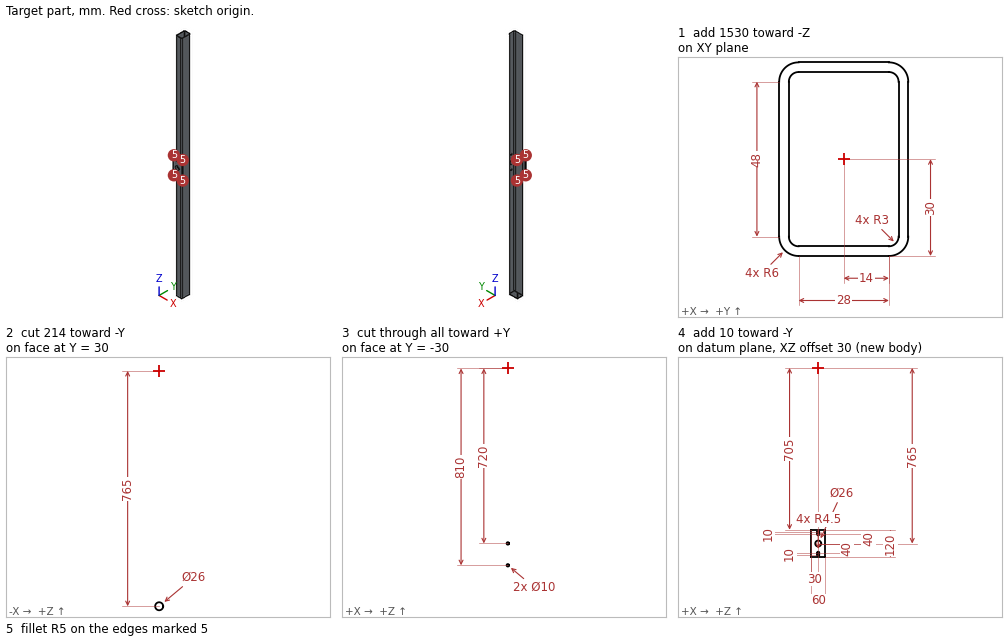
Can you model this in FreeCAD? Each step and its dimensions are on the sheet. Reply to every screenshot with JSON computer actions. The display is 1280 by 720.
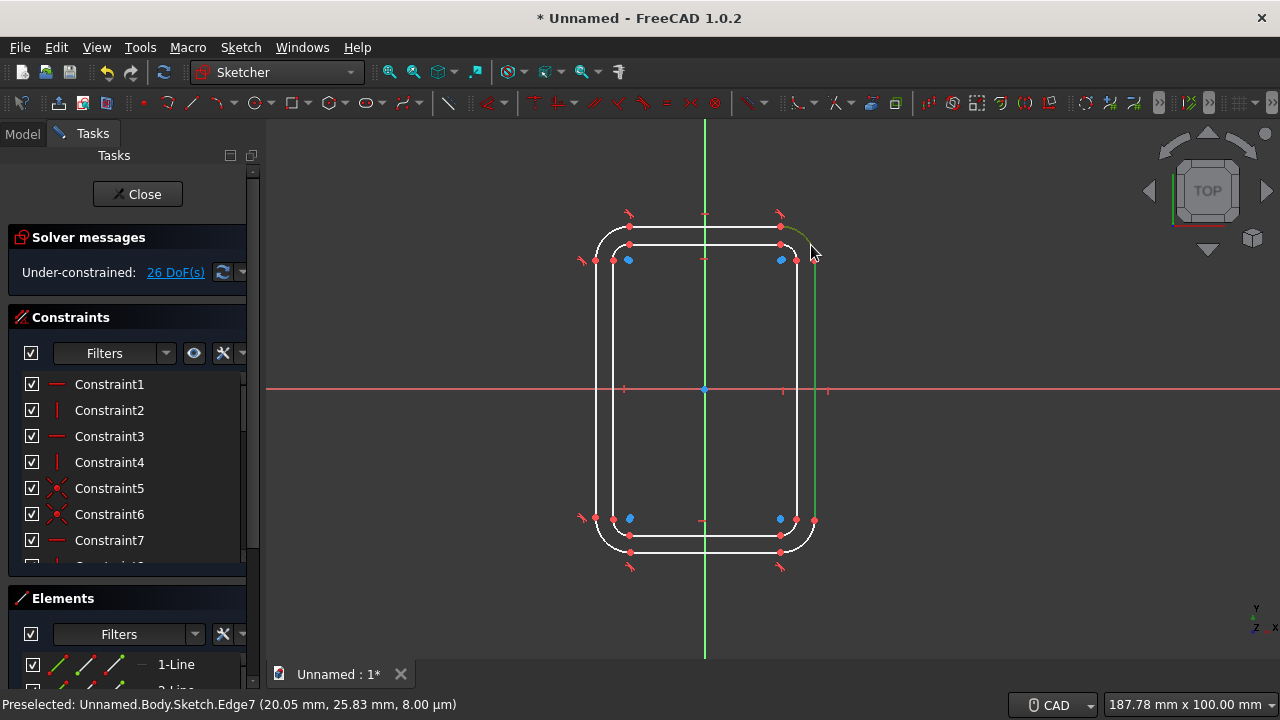
{"action": "left_click", "coordinate": [644, 104]}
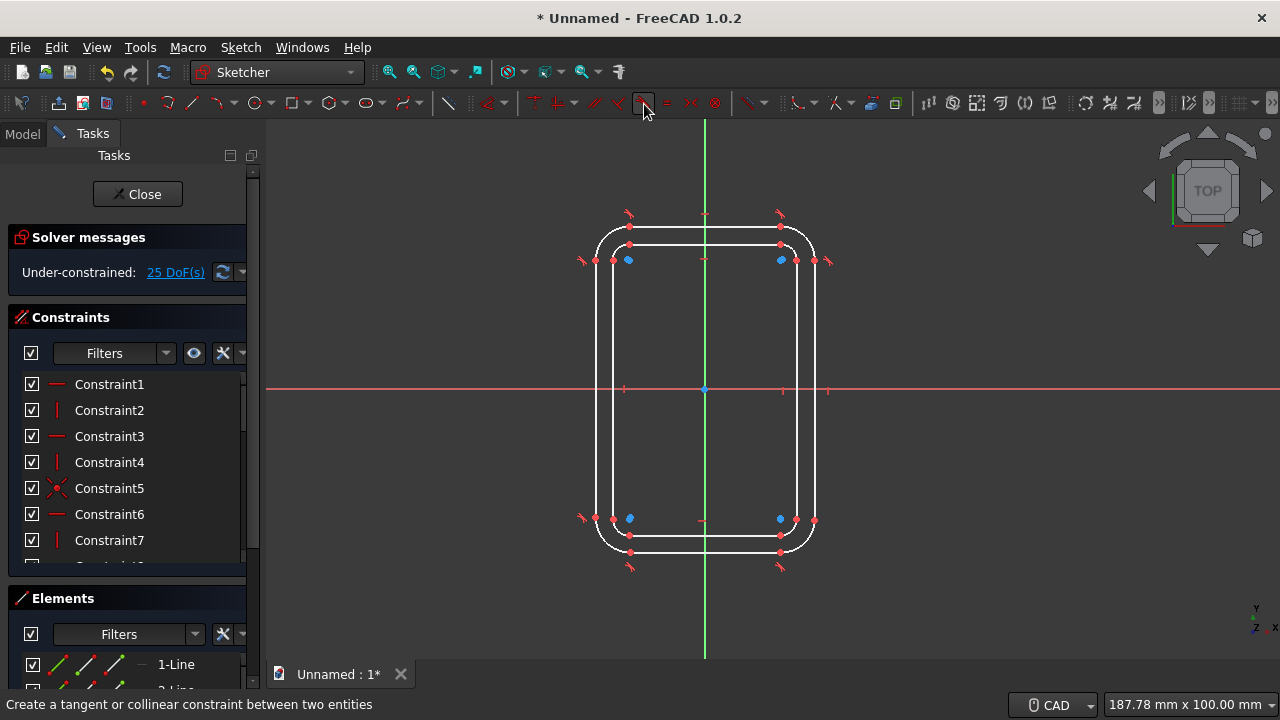
{"action": "left_click", "coordinate": [815, 339]}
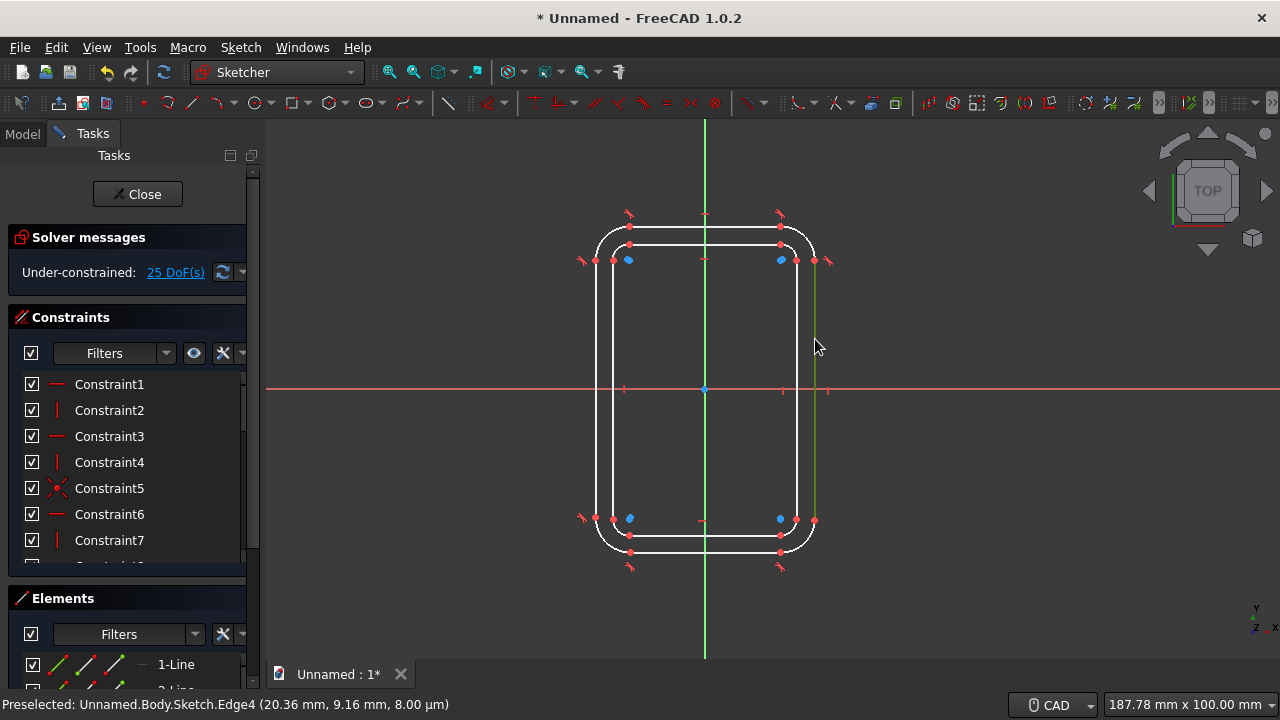
{"action": "left_click", "coordinate": [796, 549]}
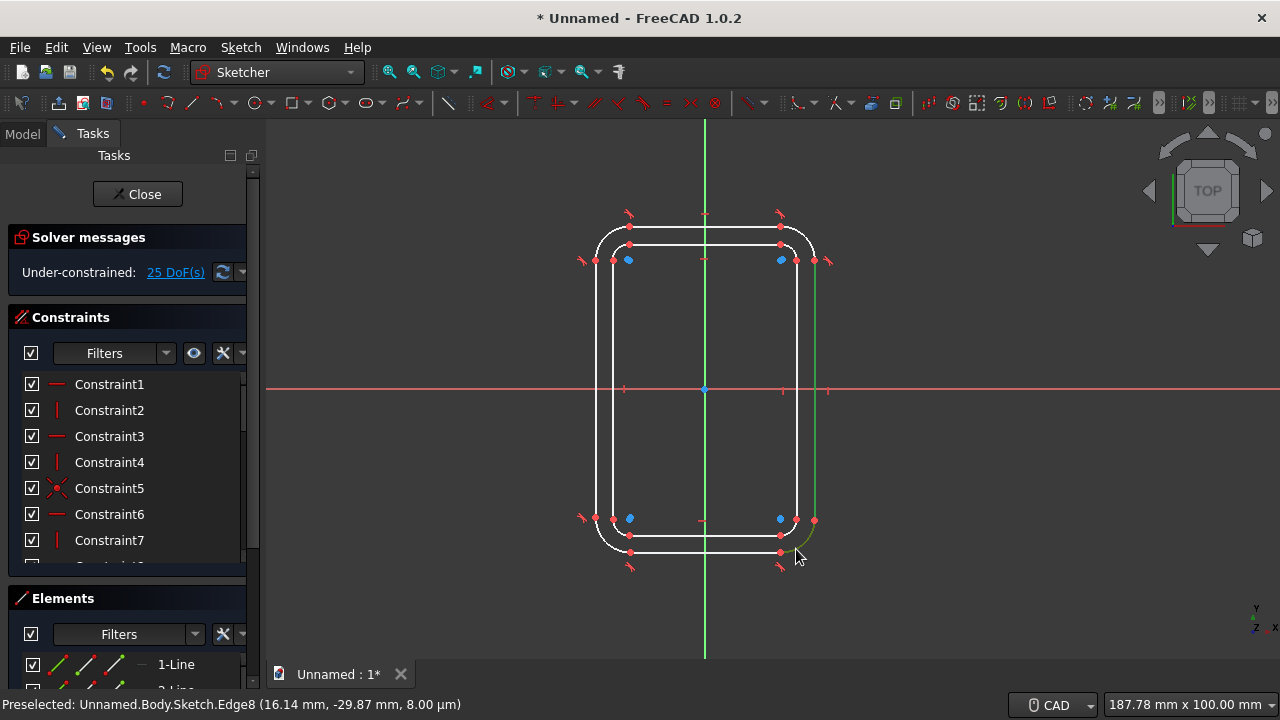
{"action": "left_click", "coordinate": [644, 104]}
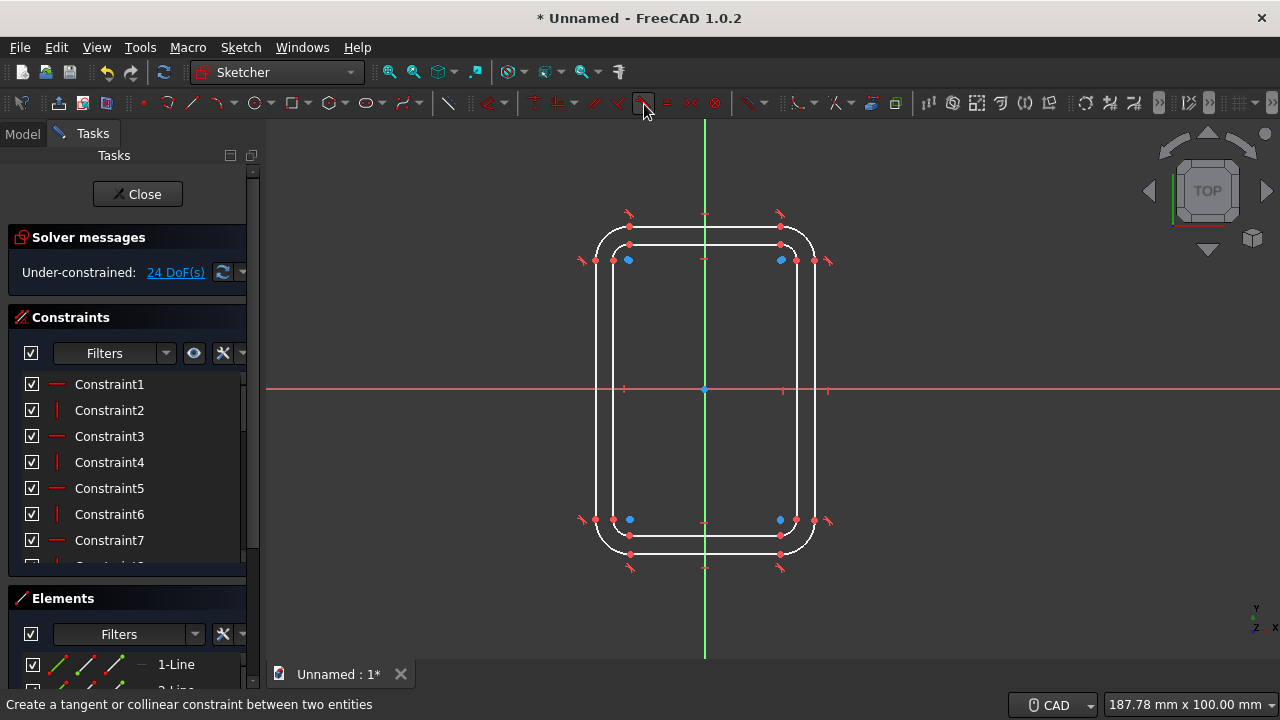
{"action": "left_click", "coordinate": [675, 536]}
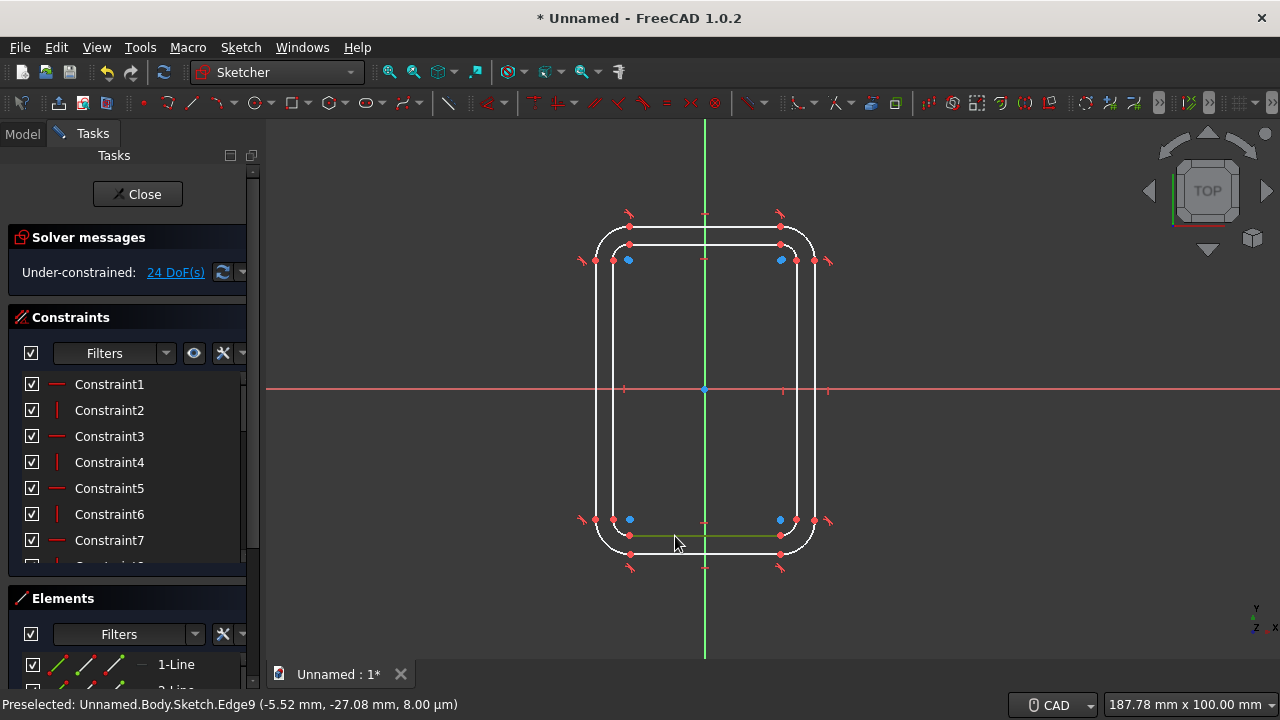
{"action": "left_click", "coordinate": [792, 531]}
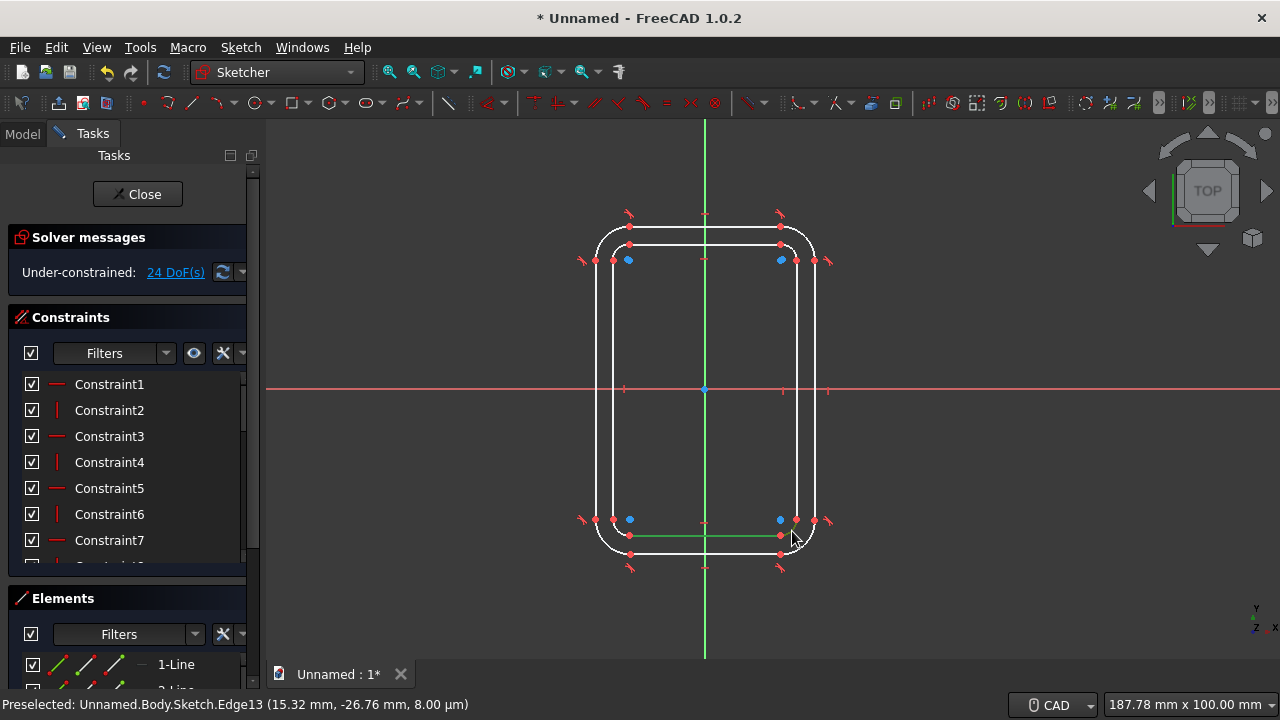
{"action": "left_click", "coordinate": [644, 104]}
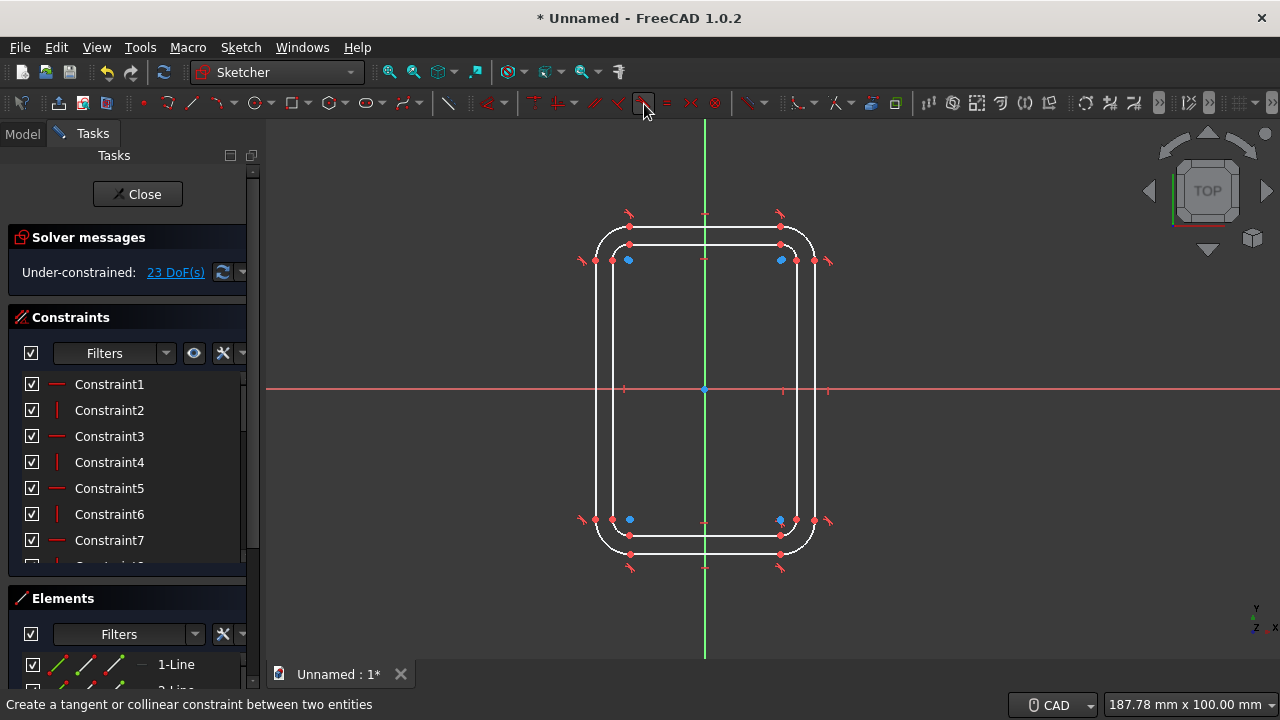
{"action": "left_click", "coordinate": [675, 536]}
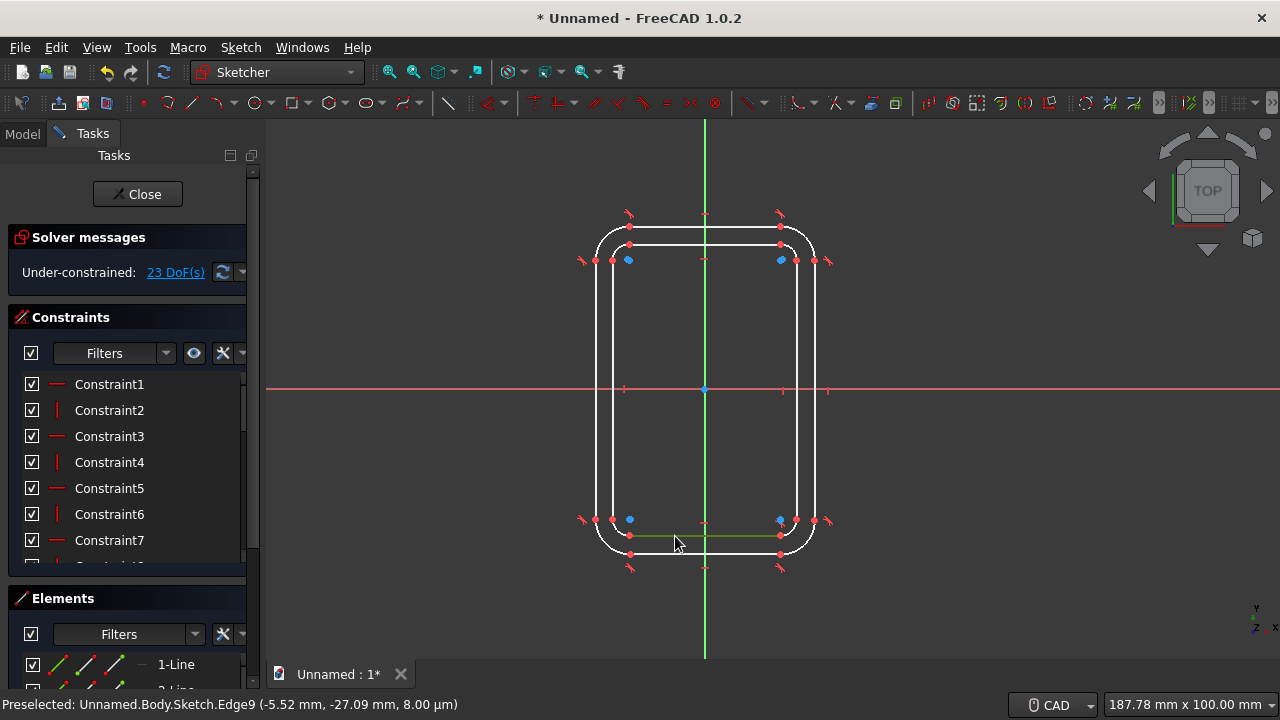
{"action": "left_click", "coordinate": [618, 531]}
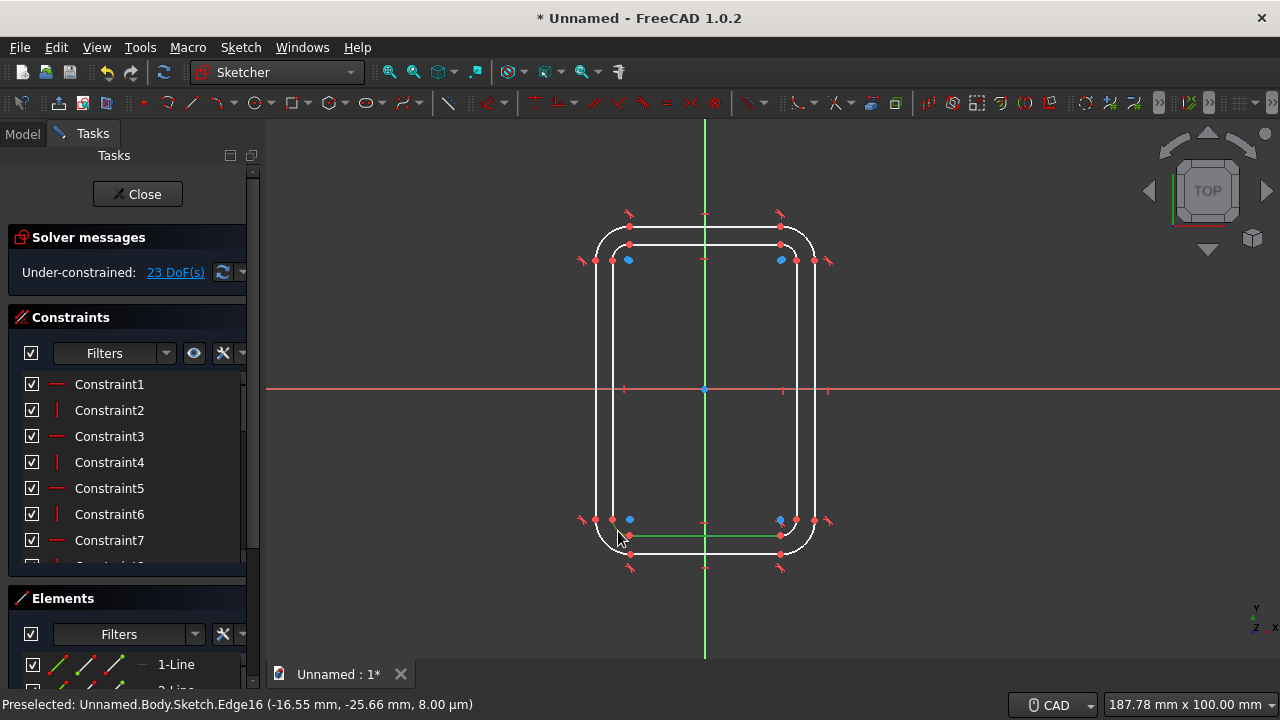
{"action": "left_click", "coordinate": [644, 104]}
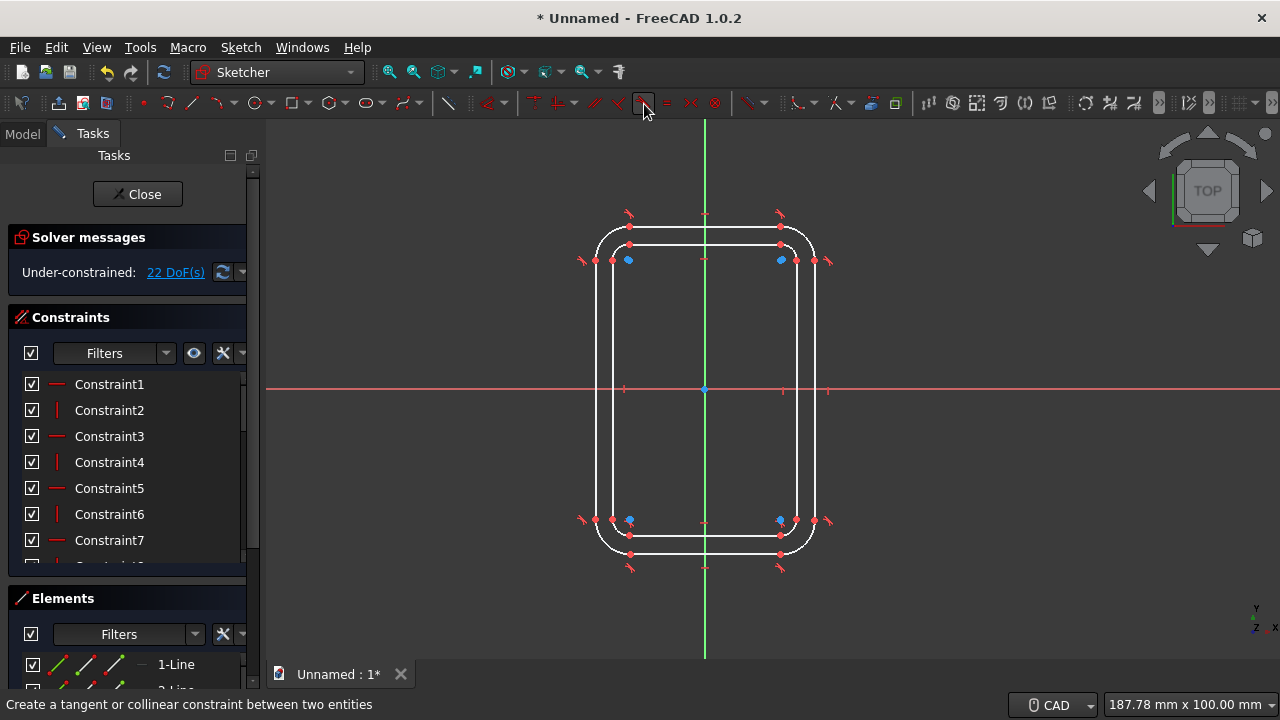
{"action": "left_click", "coordinate": [797, 442]}